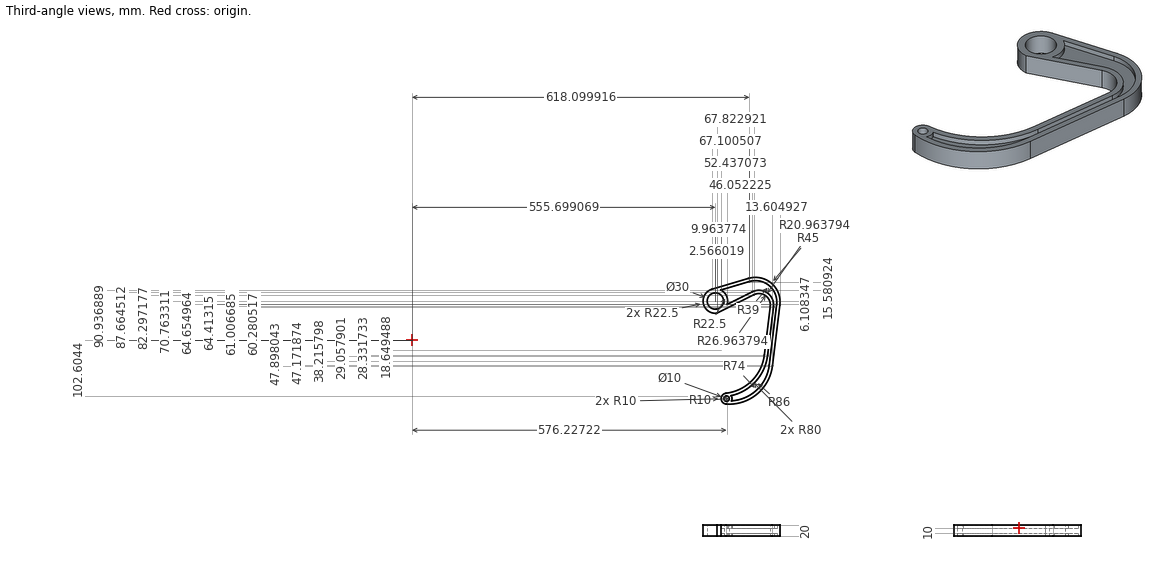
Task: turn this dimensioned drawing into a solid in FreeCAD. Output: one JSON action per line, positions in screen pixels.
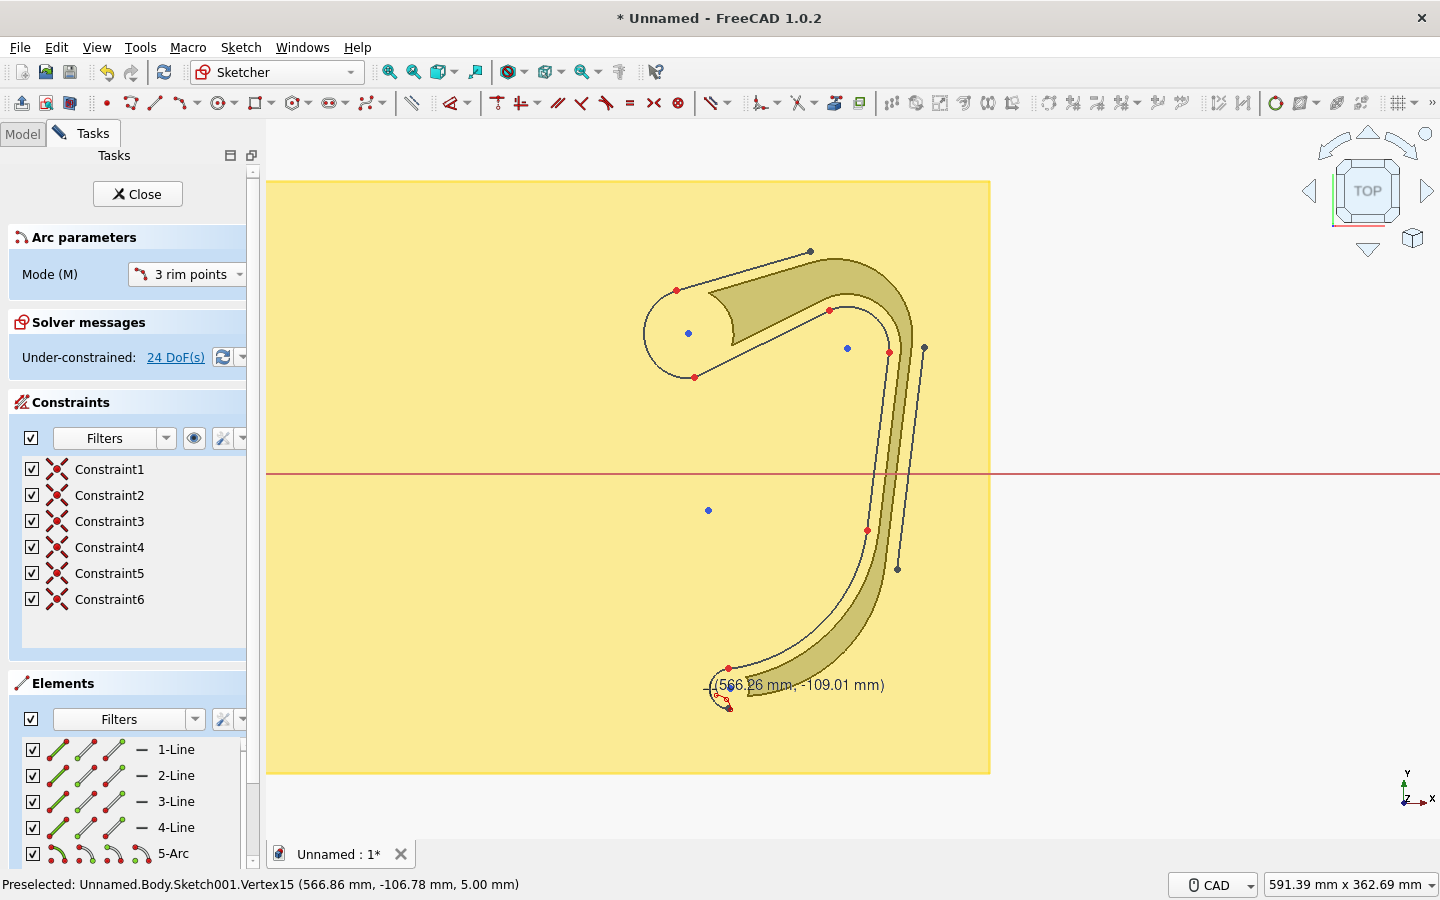
{"action": "left_click", "coordinate": [728, 709]}
{"action": "left_click", "coordinate": [897, 570]}
{"action": "left_click", "coordinate": [840, 672]}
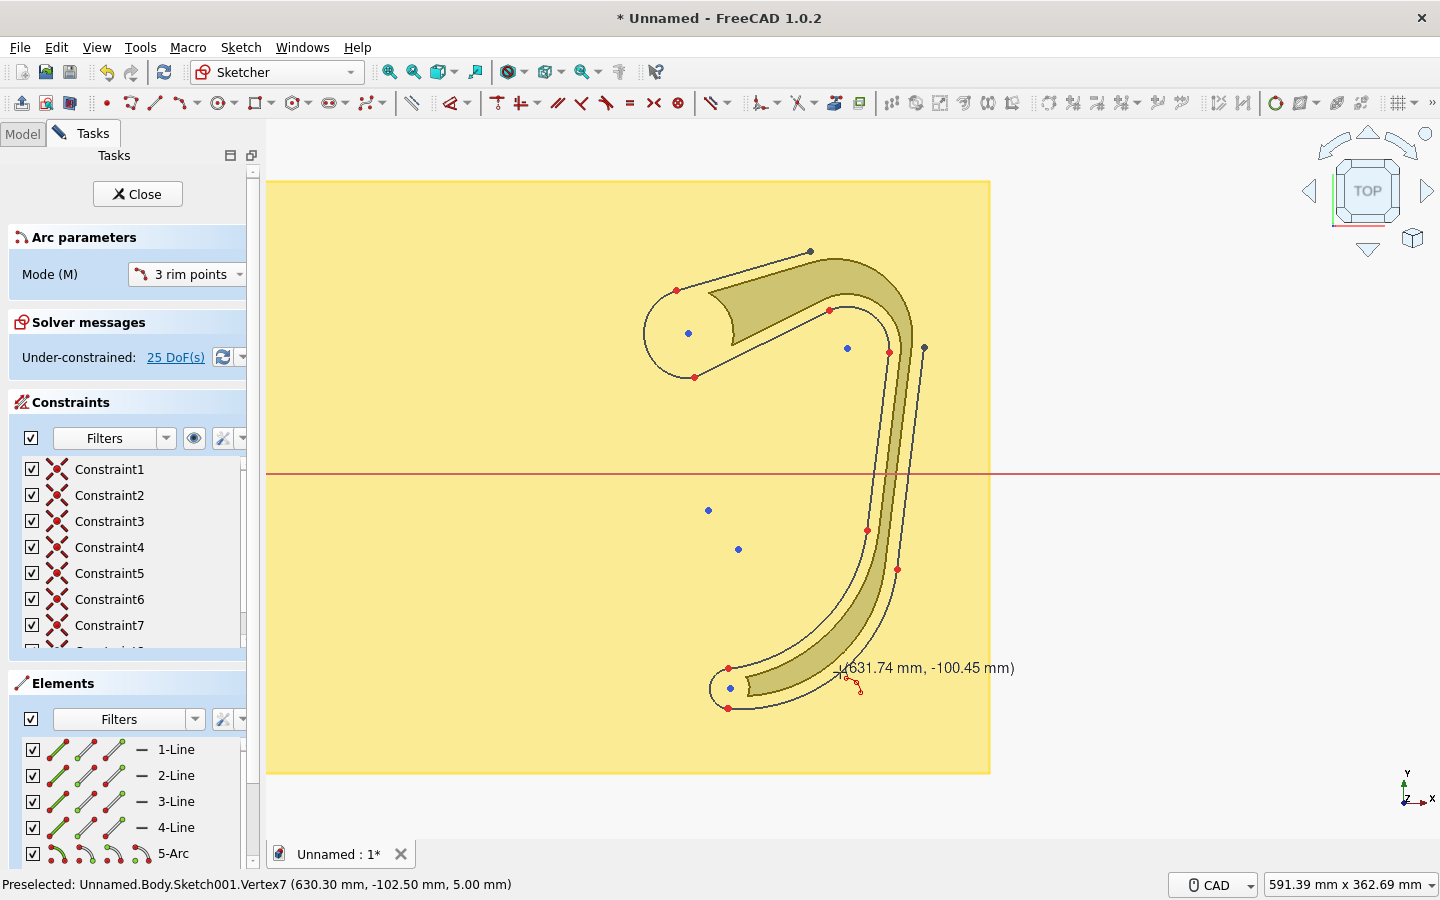
{"action": "left_click", "coordinate": [924, 348]}
{"action": "left_click", "coordinate": [810, 252]}
{"action": "left_click", "coordinate": [893, 268]}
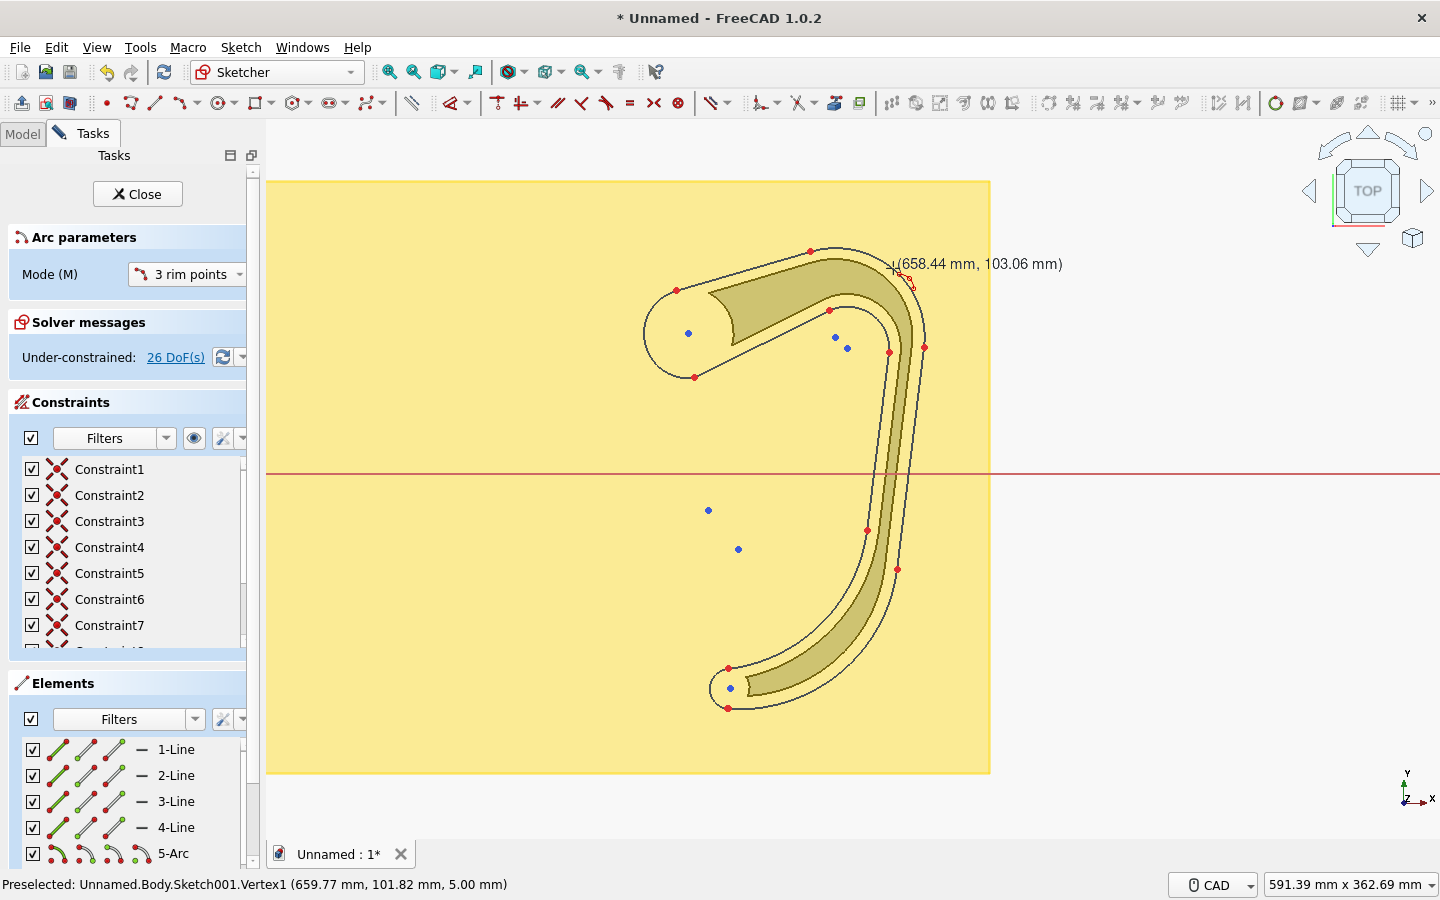
{"action": "left_click", "coordinate": [156, 104]}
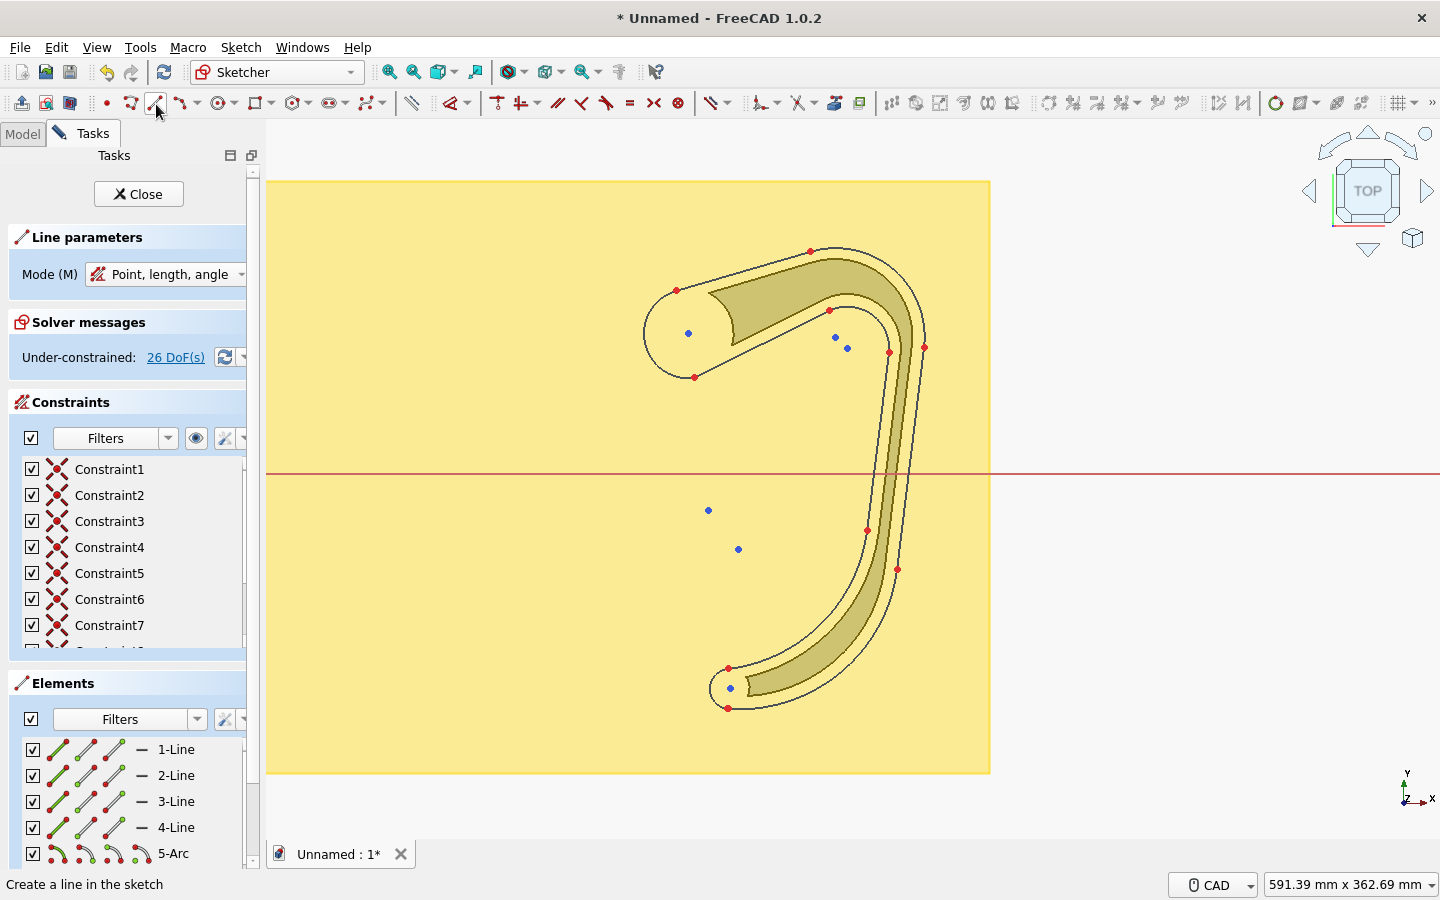
{"action": "scroll", "coordinate": [709, 293], "scroll_direction": "up", "scroll_amount": 2}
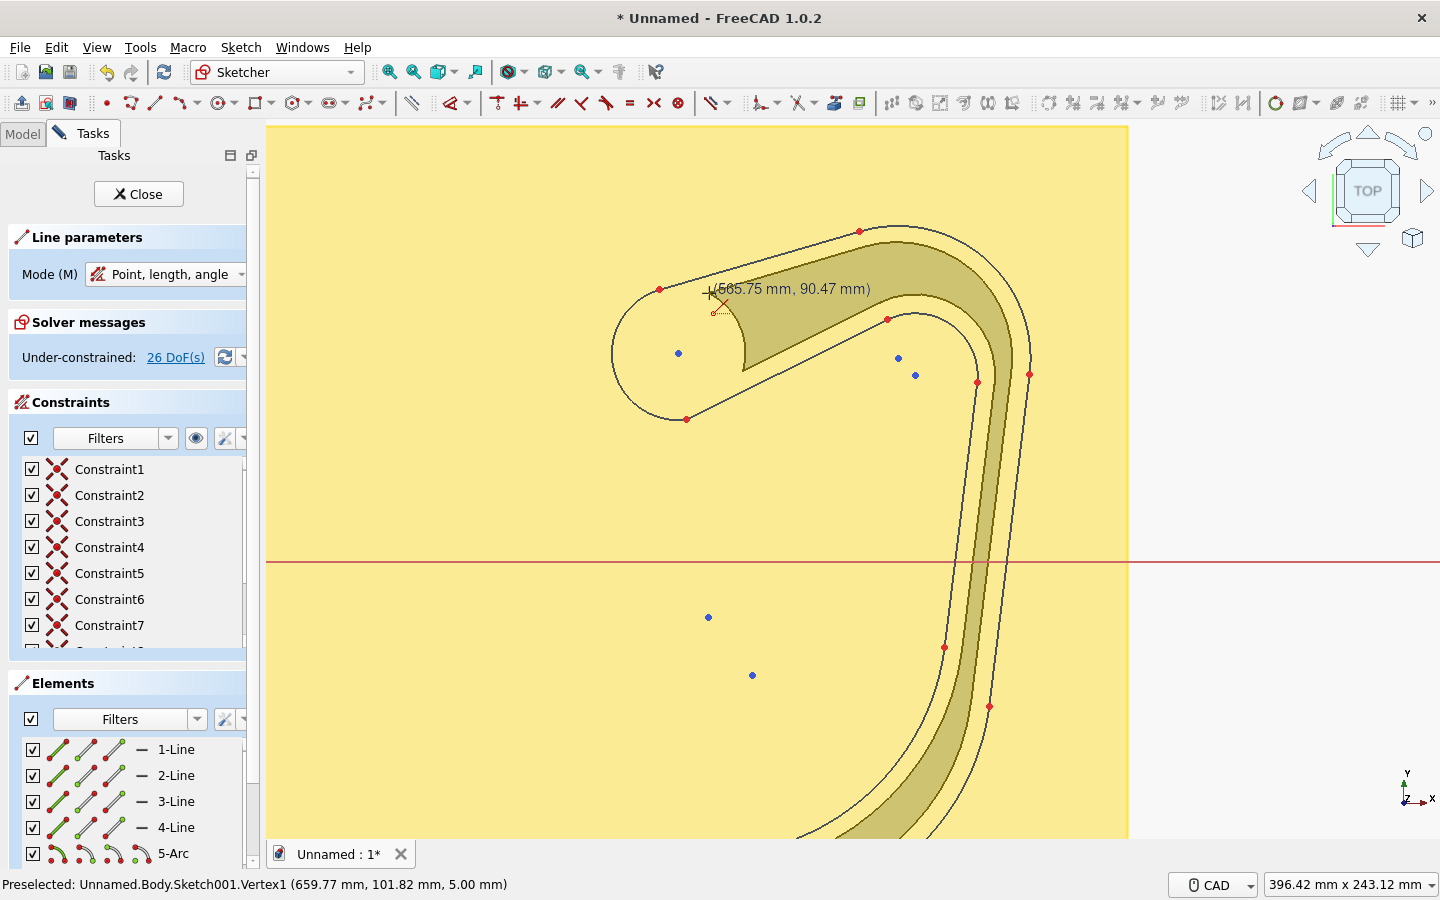
{"action": "left_click", "coordinate": [709, 293]}
{"action": "left_click", "coordinate": [864, 247]}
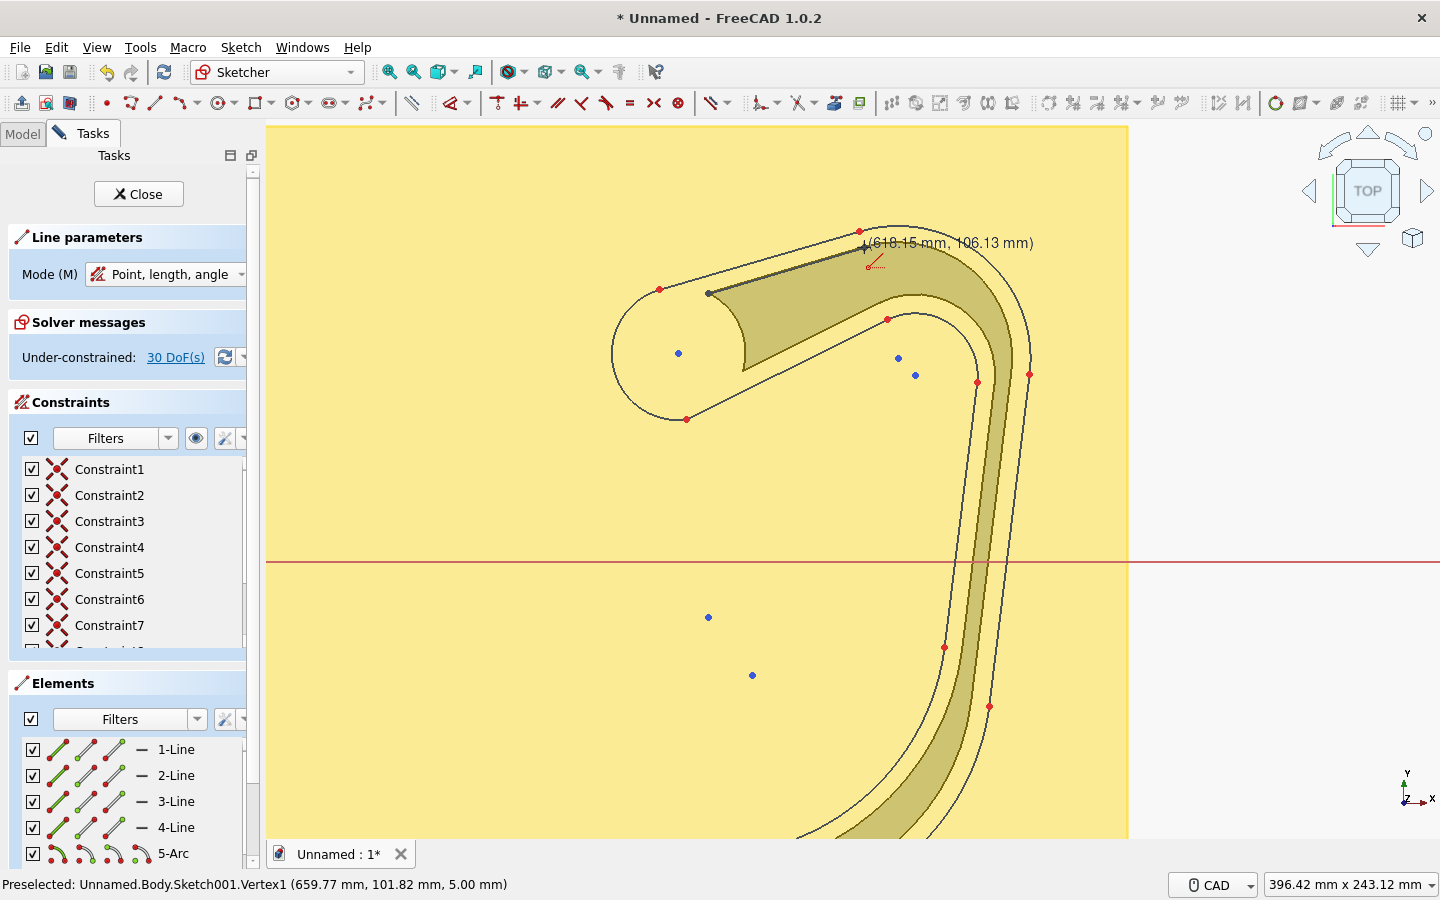
{"action": "left_click", "coordinate": [1011, 372]}
{"action": "left_click", "coordinate": [971, 702]}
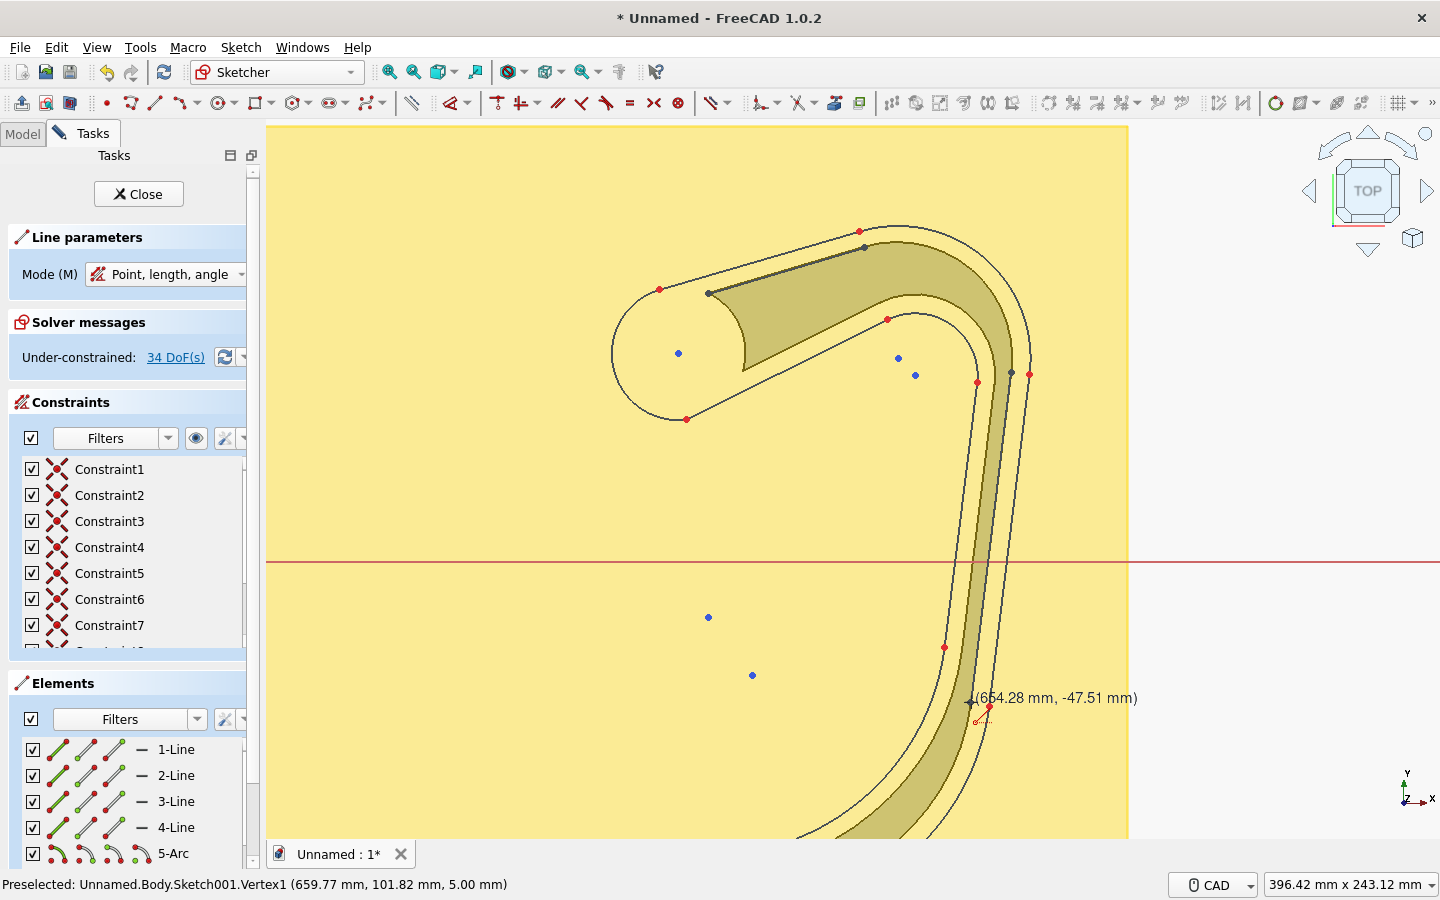
{"action": "left_click", "coordinate": [962, 648]}
{"action": "left_click", "coordinate": [995, 384]}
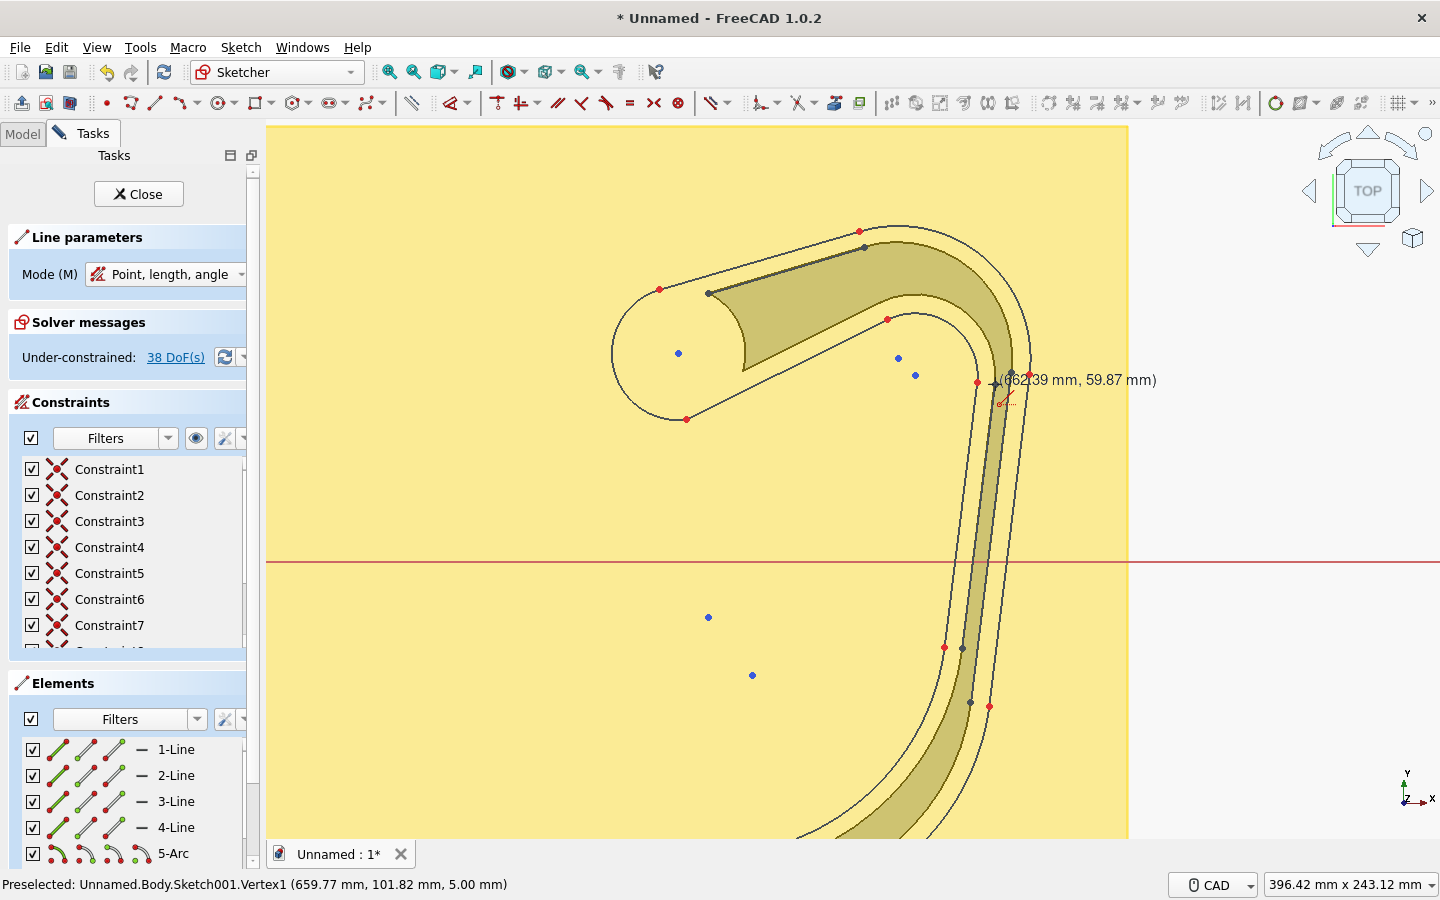
{"action": "left_click", "coordinate": [880, 303]}
{"action": "left_click", "coordinate": [743, 371]}